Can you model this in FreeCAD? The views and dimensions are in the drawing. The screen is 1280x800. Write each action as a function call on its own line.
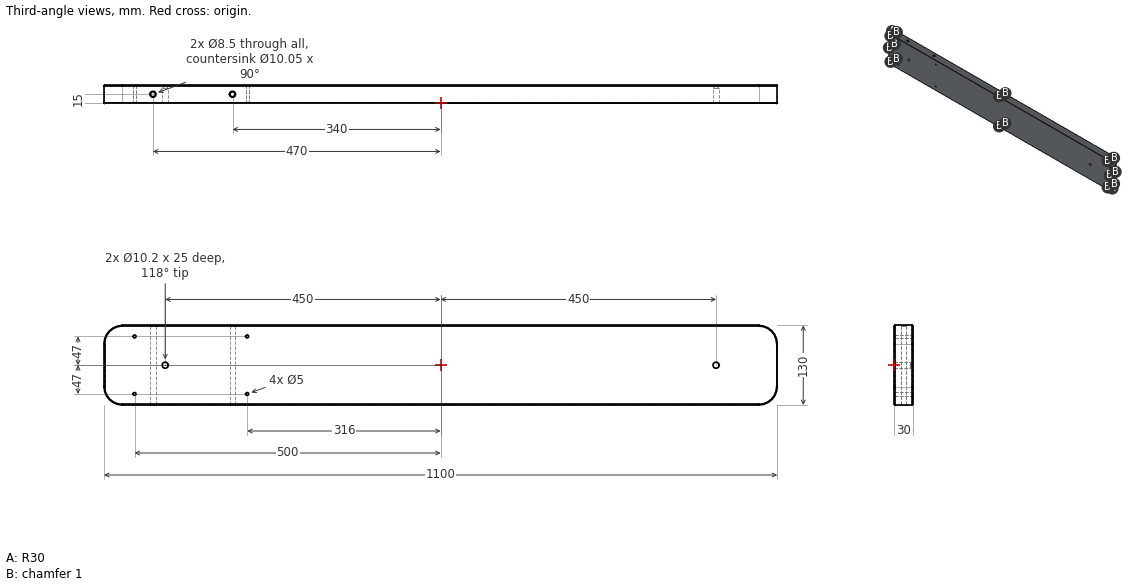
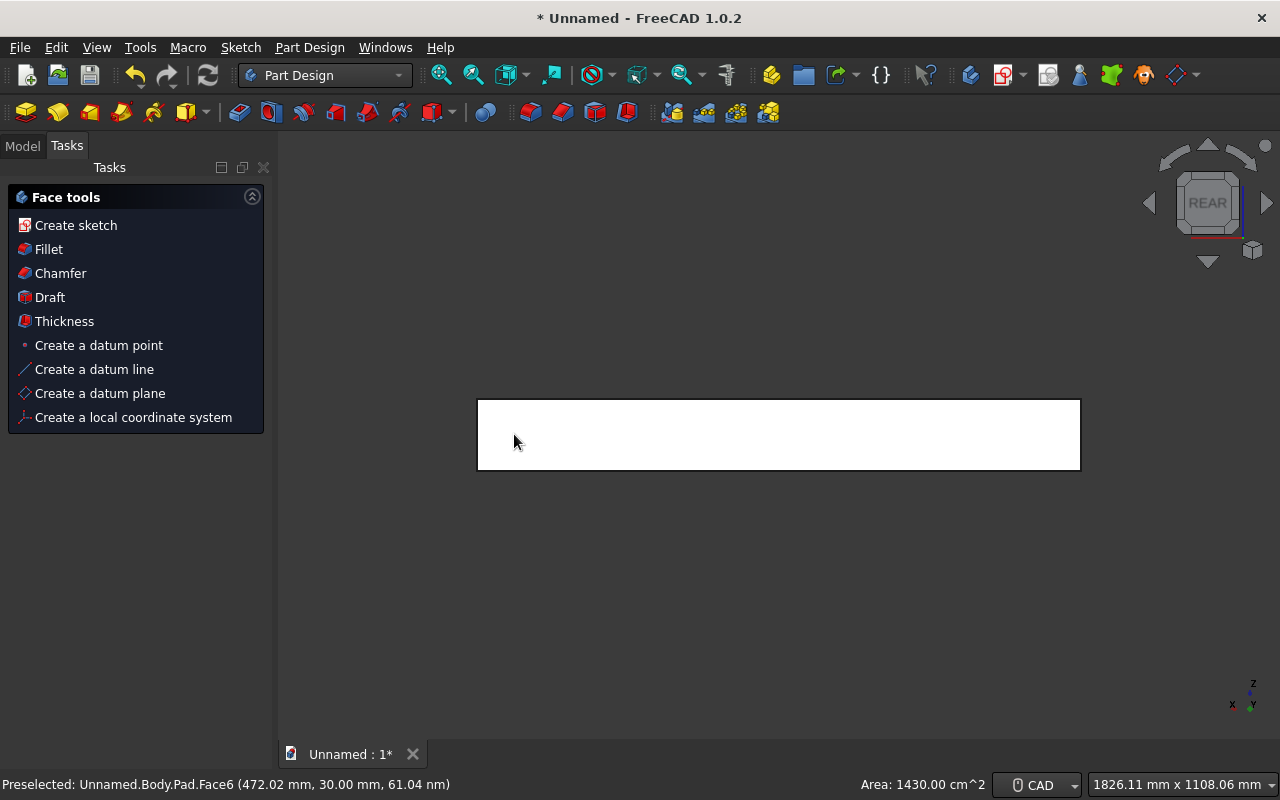
click(1004, 76)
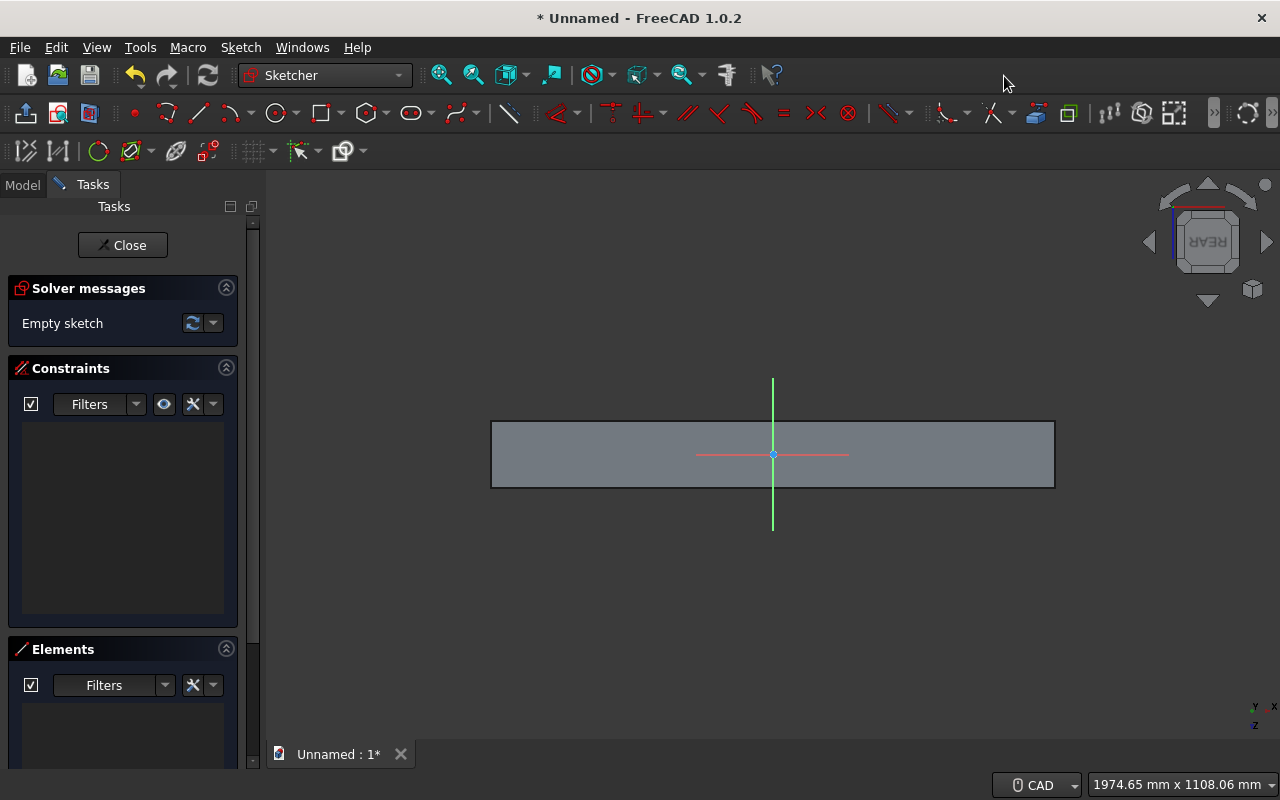
scroll(536, 454, up, 9)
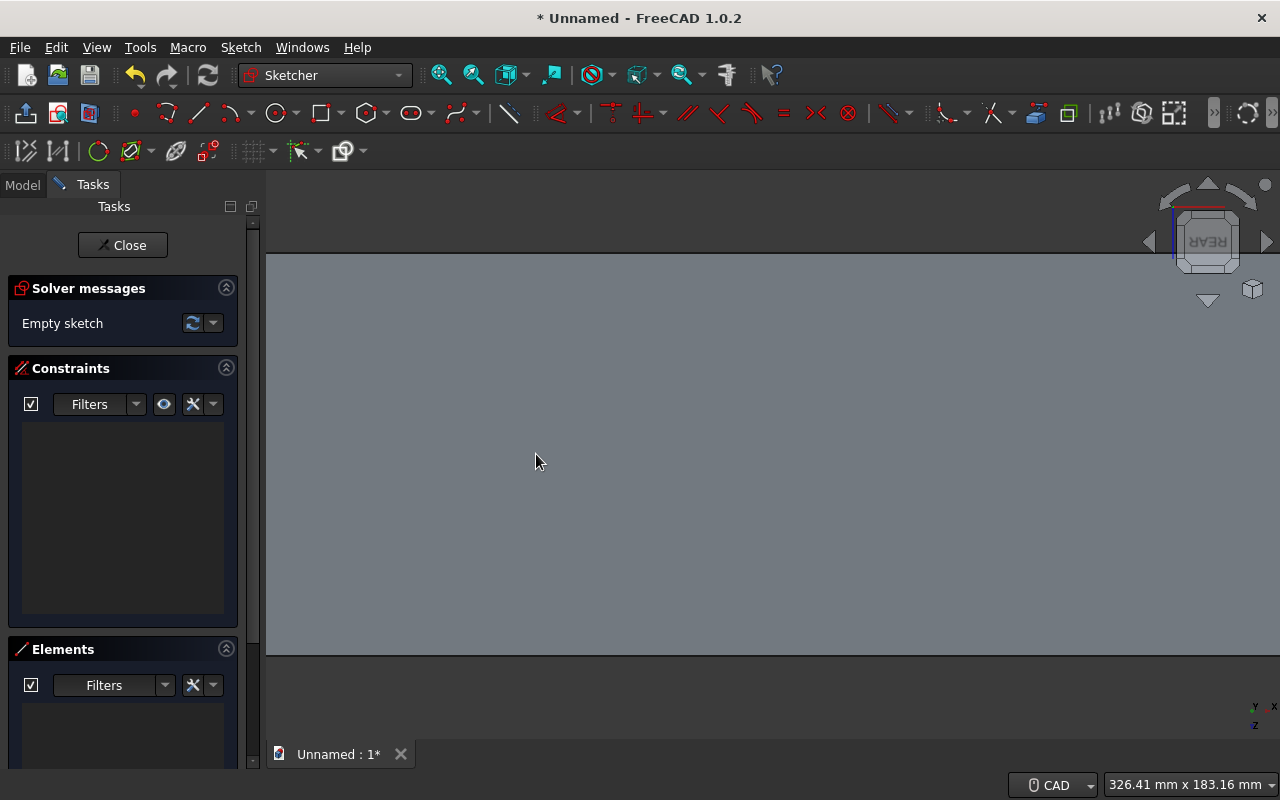
click(276, 114)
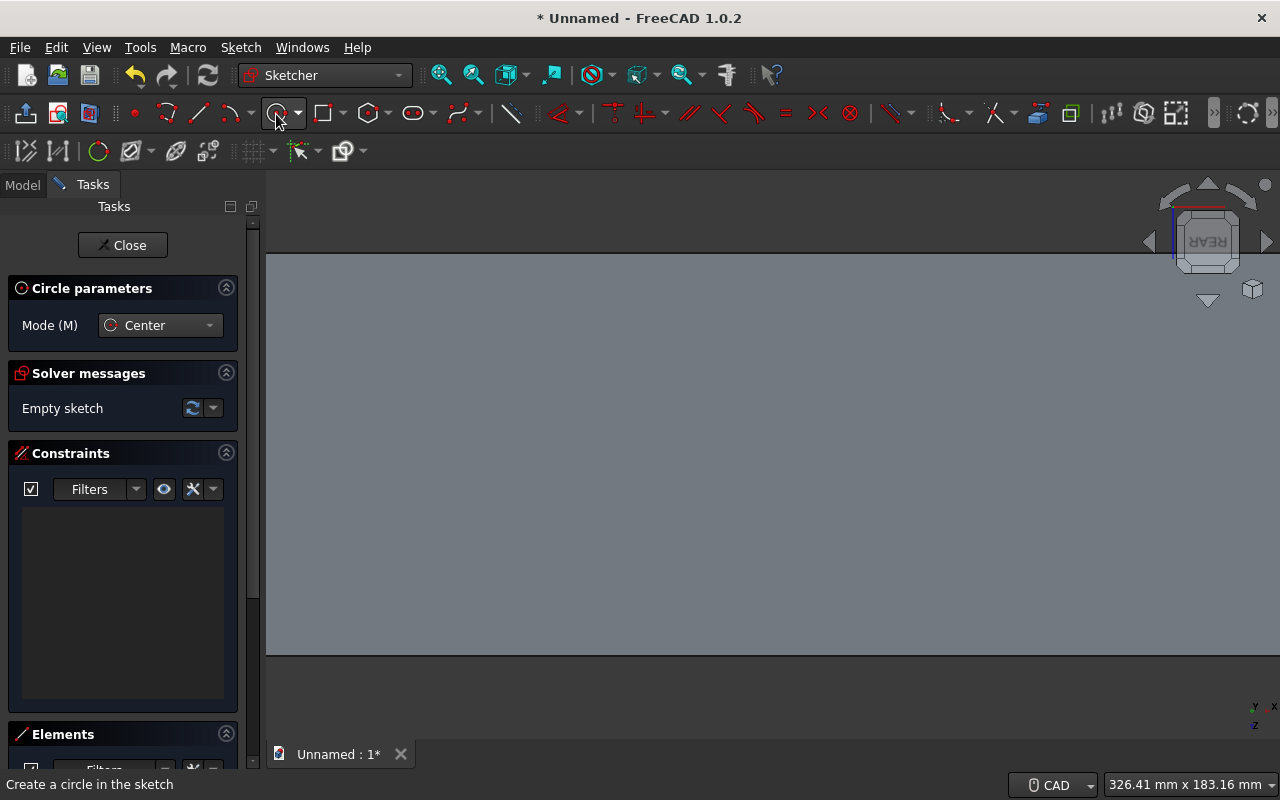
scroll(987, 308, up, 6)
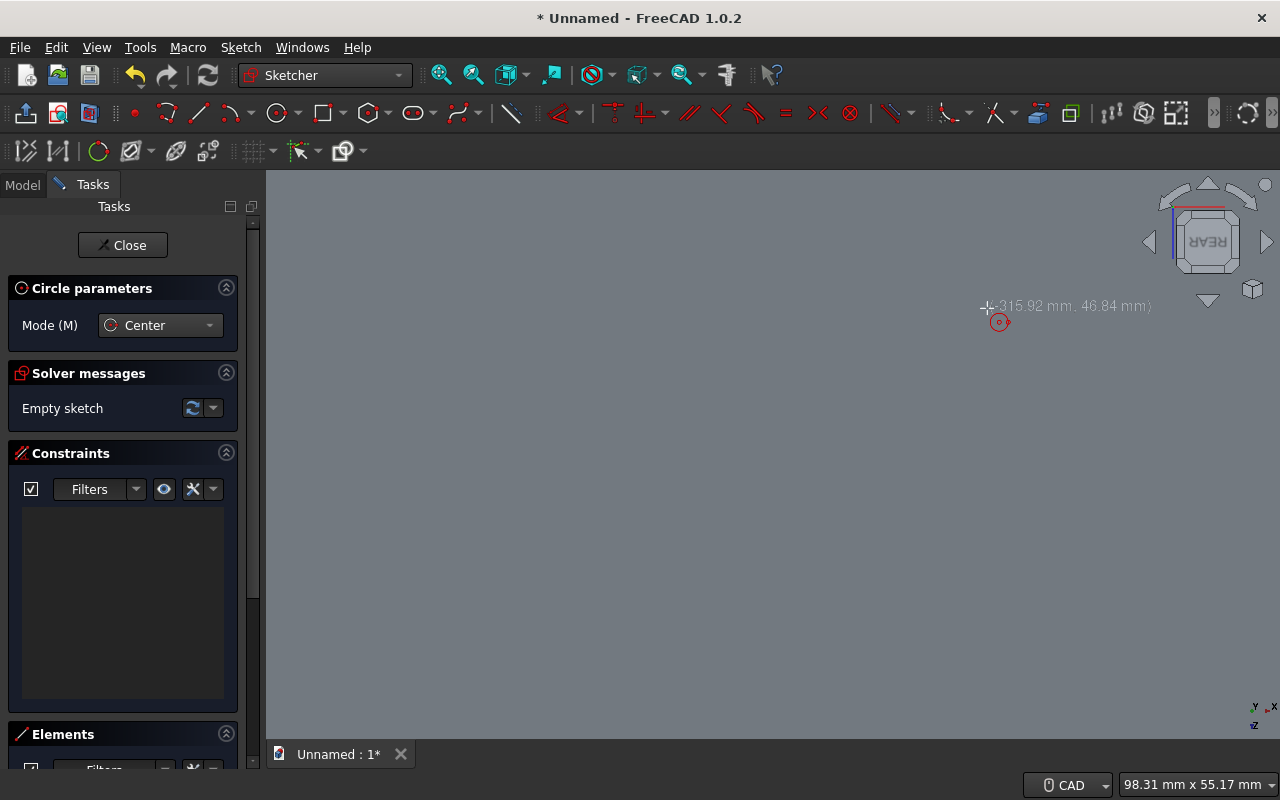
click(985, 309)
click(1003, 291)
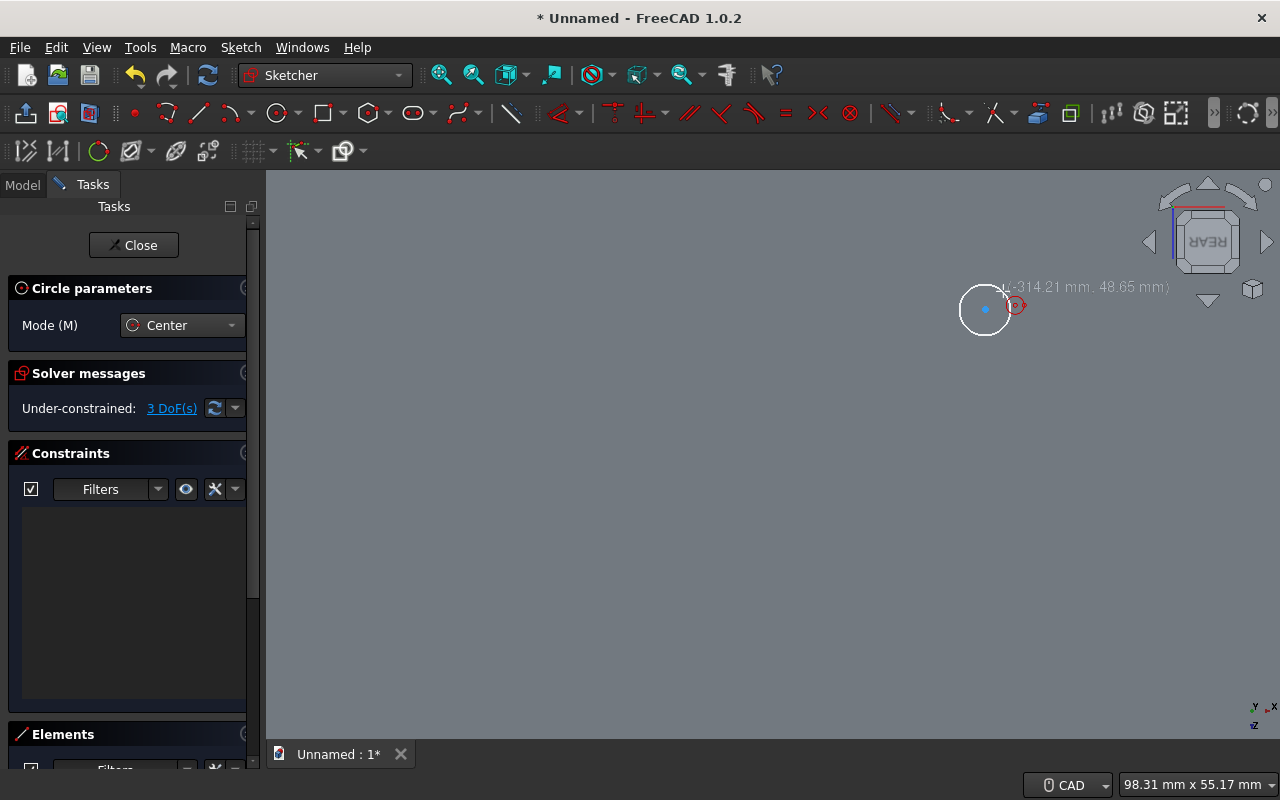
scroll(993, 308, down, 6)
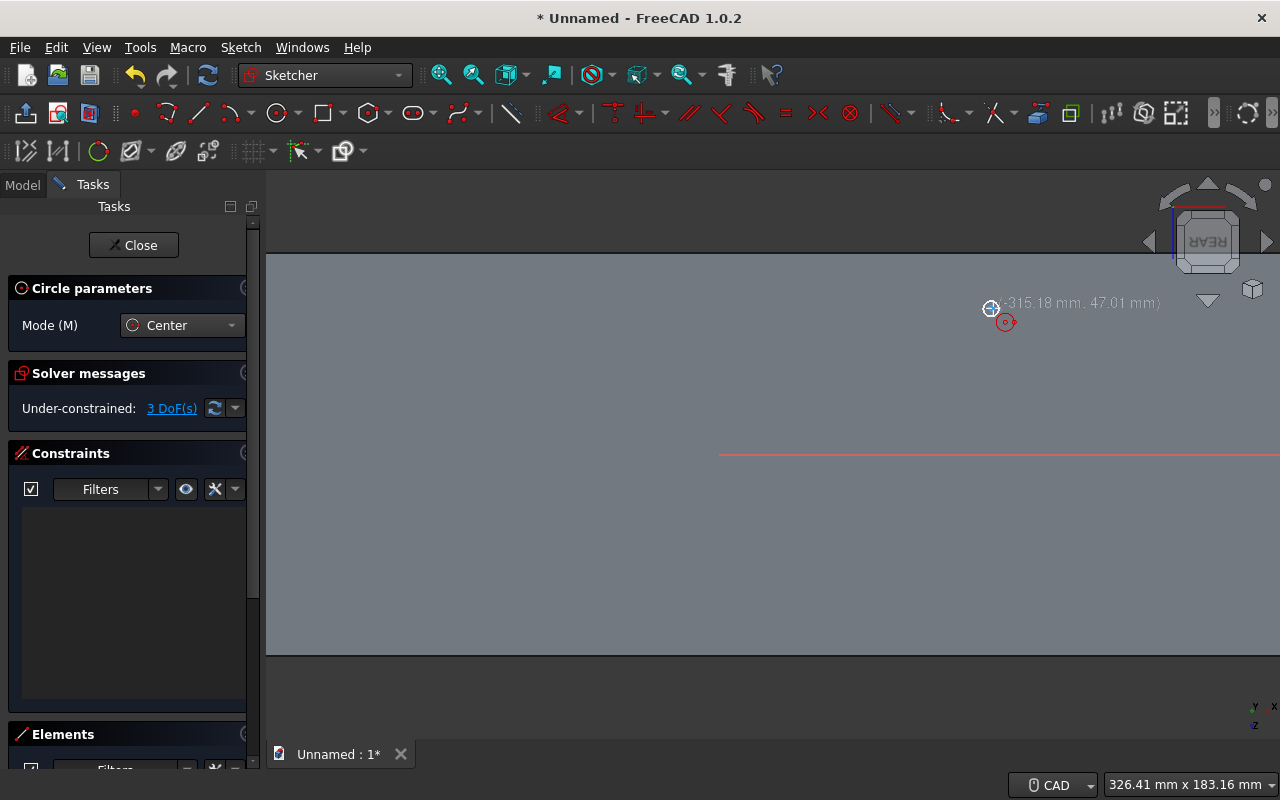
scroll(991, 601, up, 6)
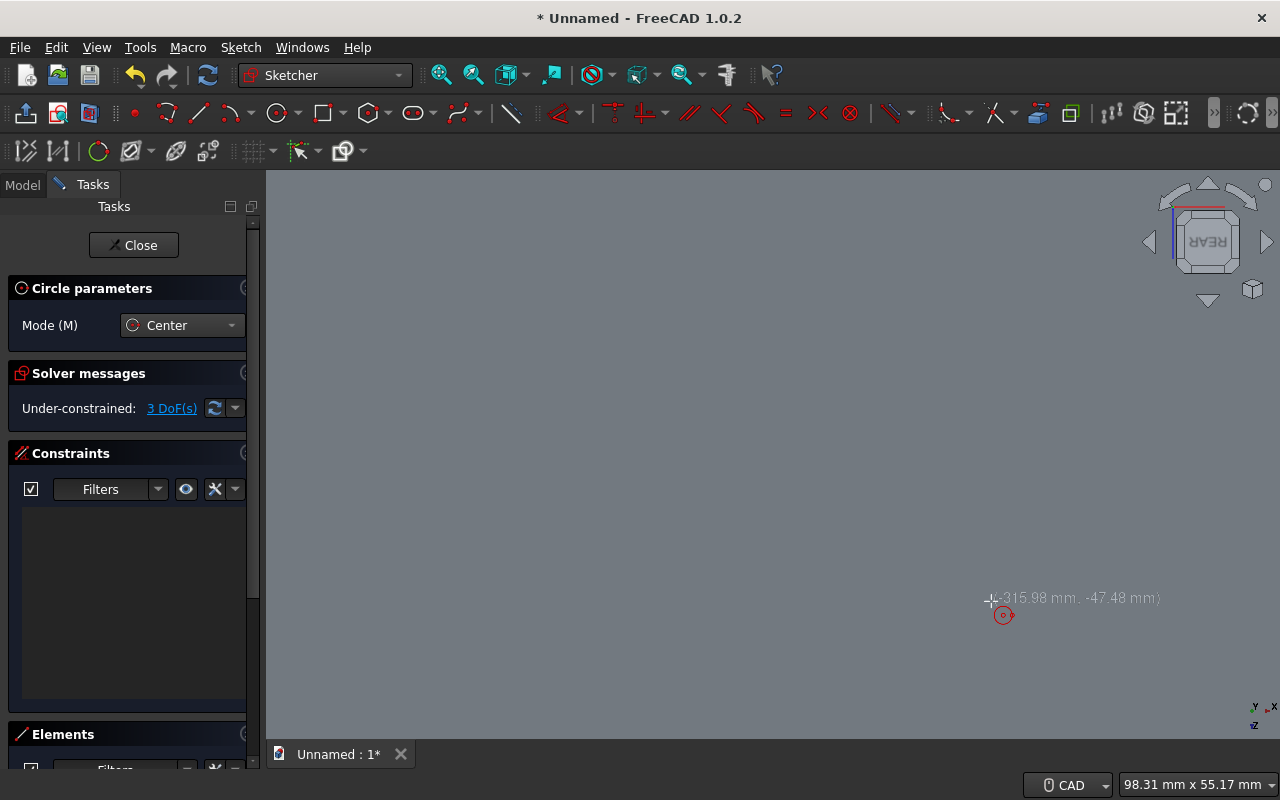
click(989, 598)
click(1007, 579)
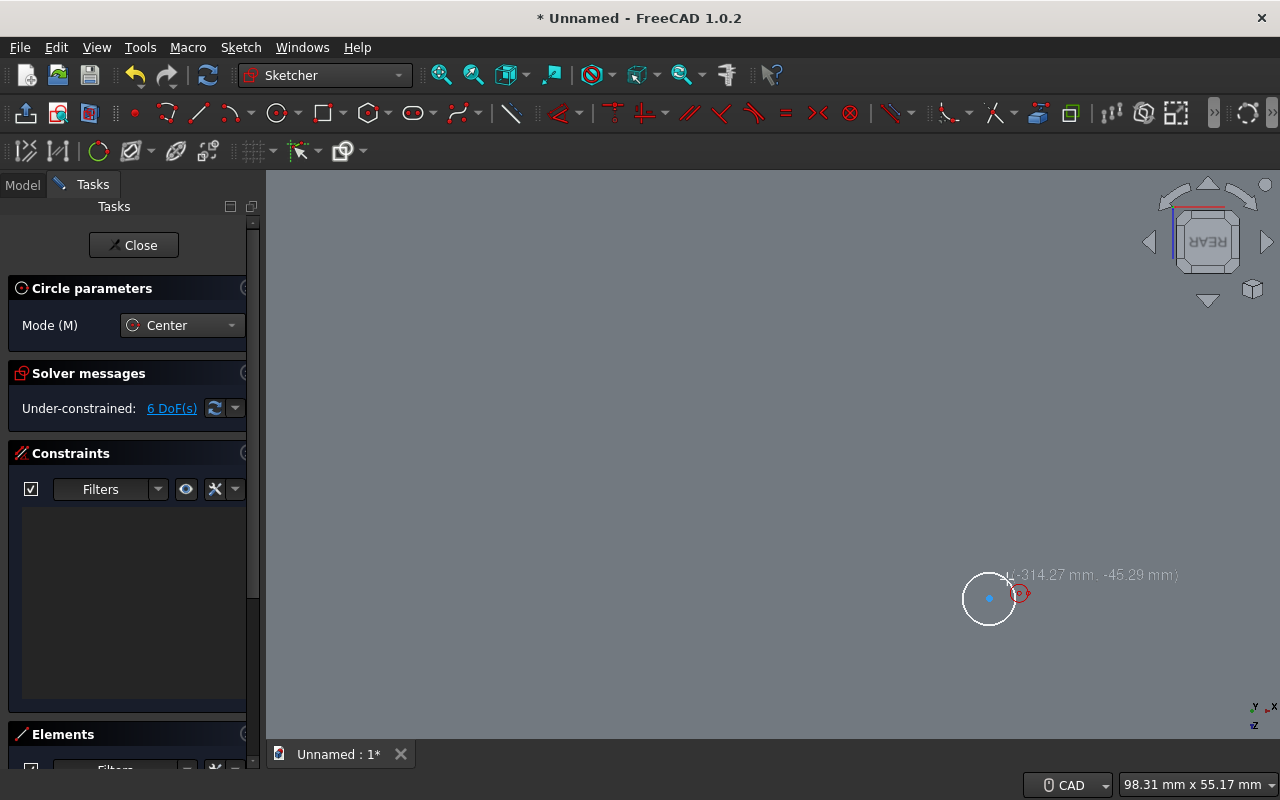
scroll(991, 602, down, 6)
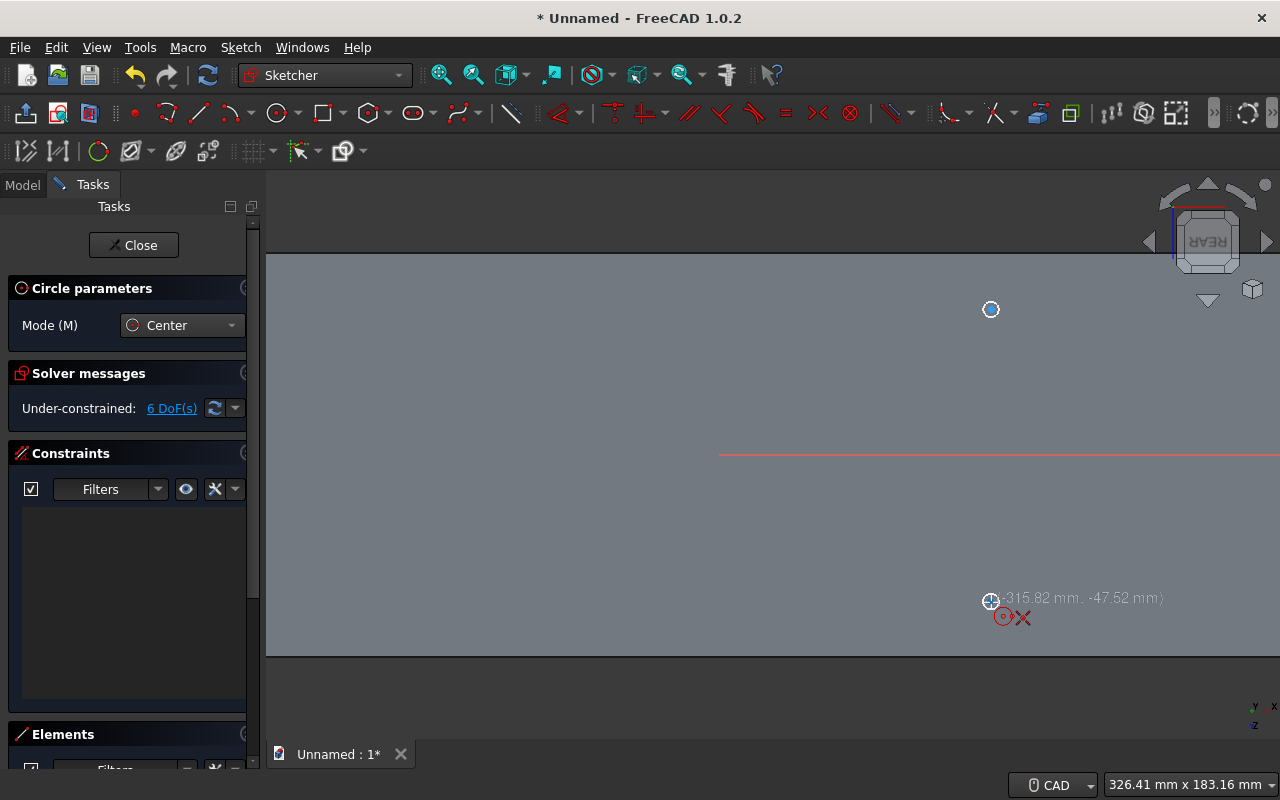
scroll(419, 309, up, 6)